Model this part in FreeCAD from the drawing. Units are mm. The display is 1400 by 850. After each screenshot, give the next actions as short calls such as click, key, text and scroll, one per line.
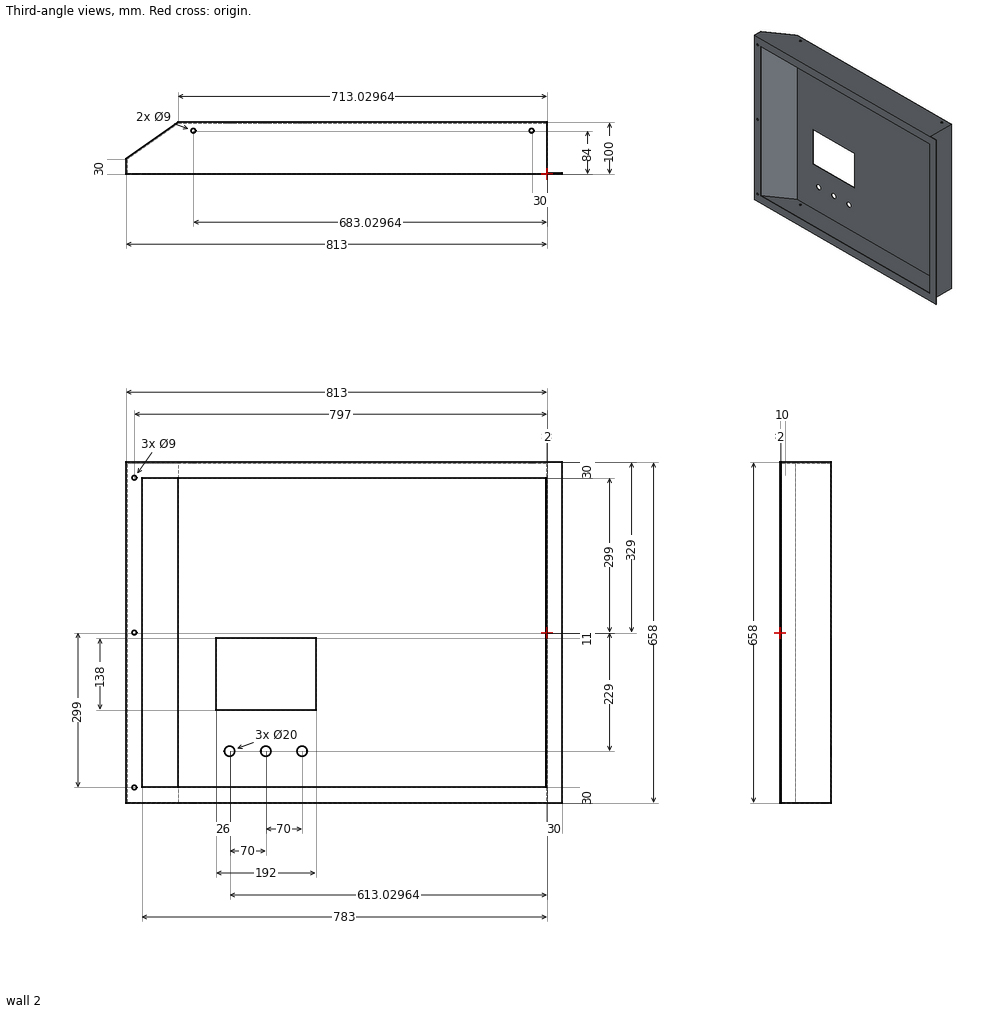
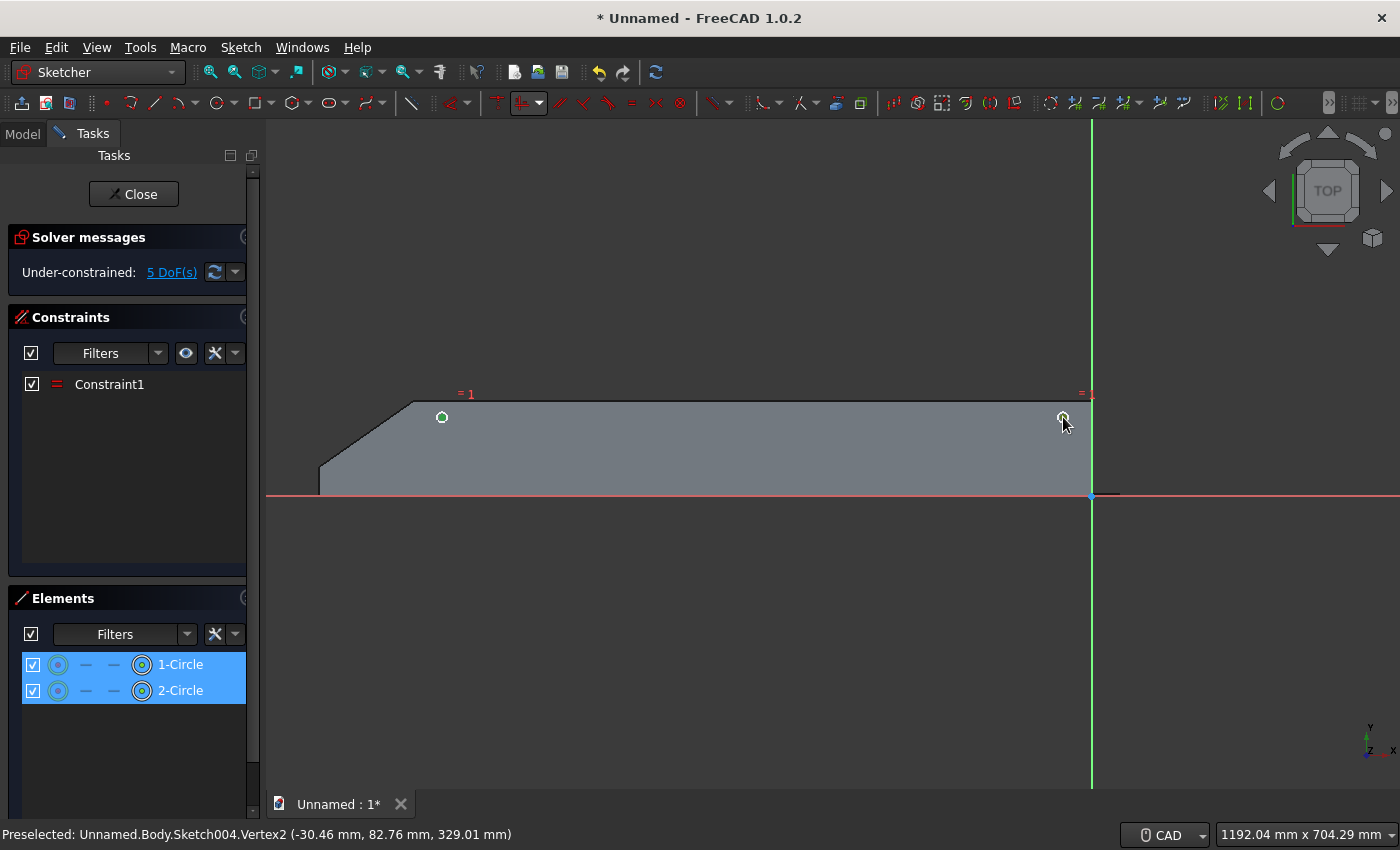
click(542, 104)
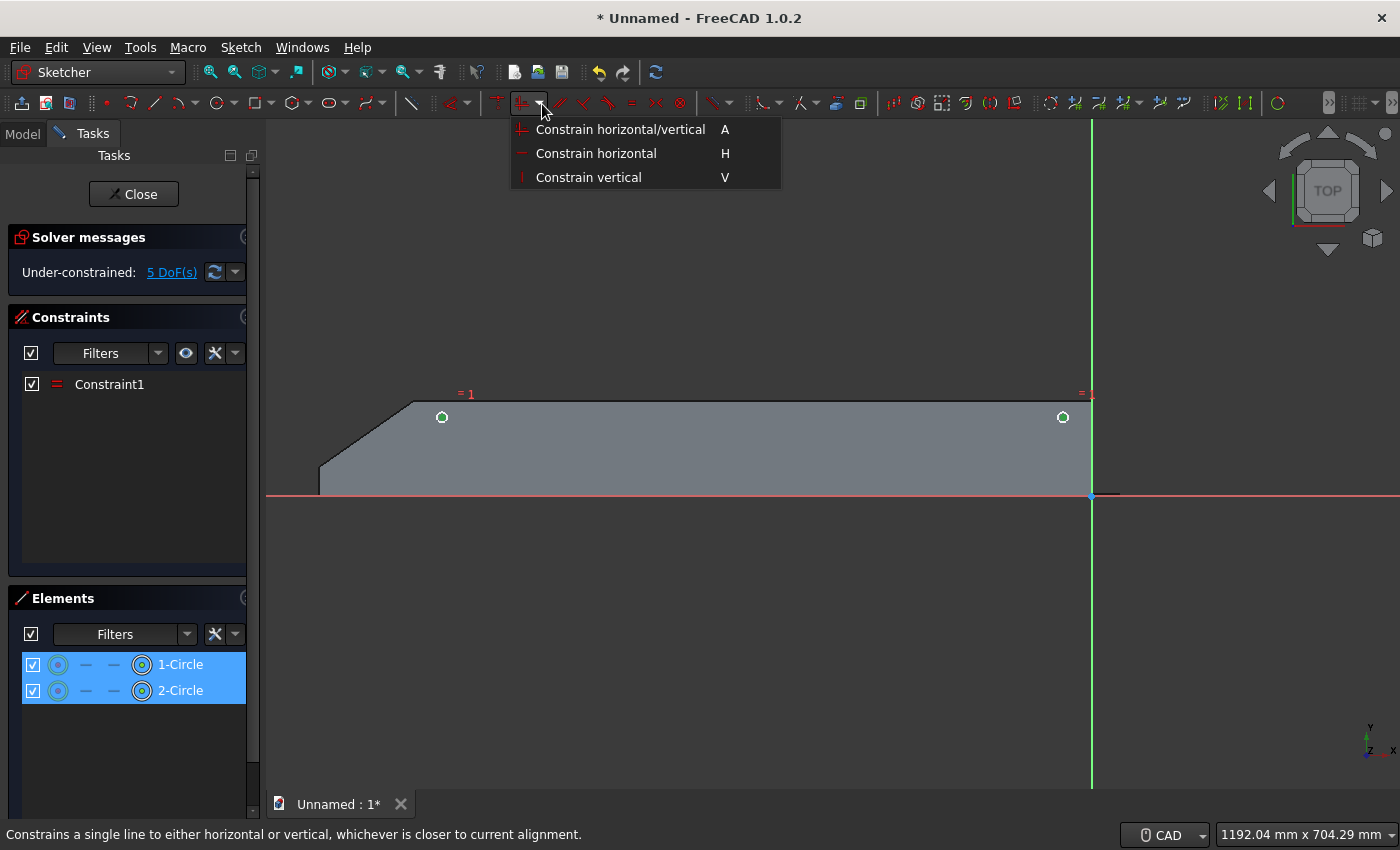
click(646, 153)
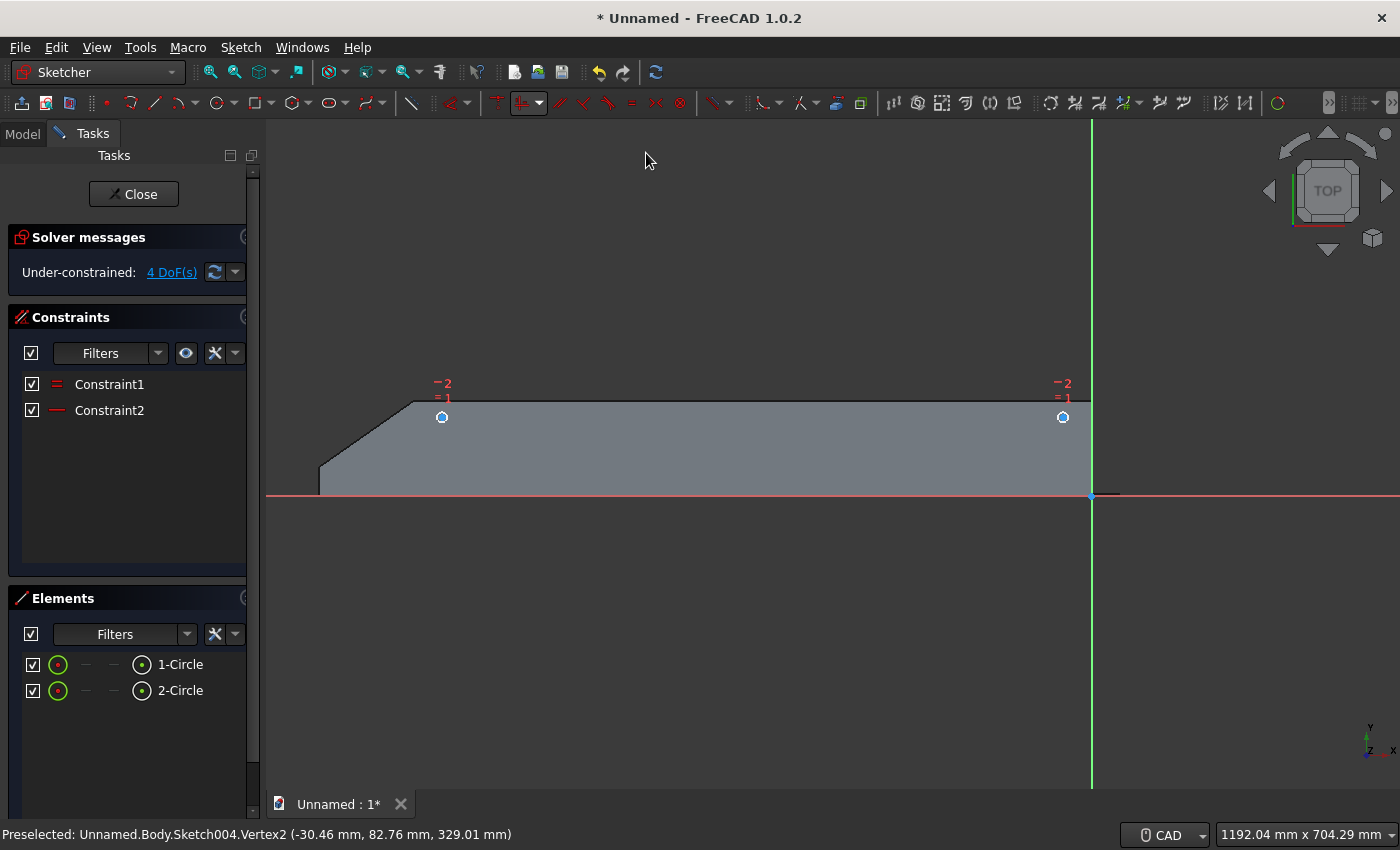
key(d)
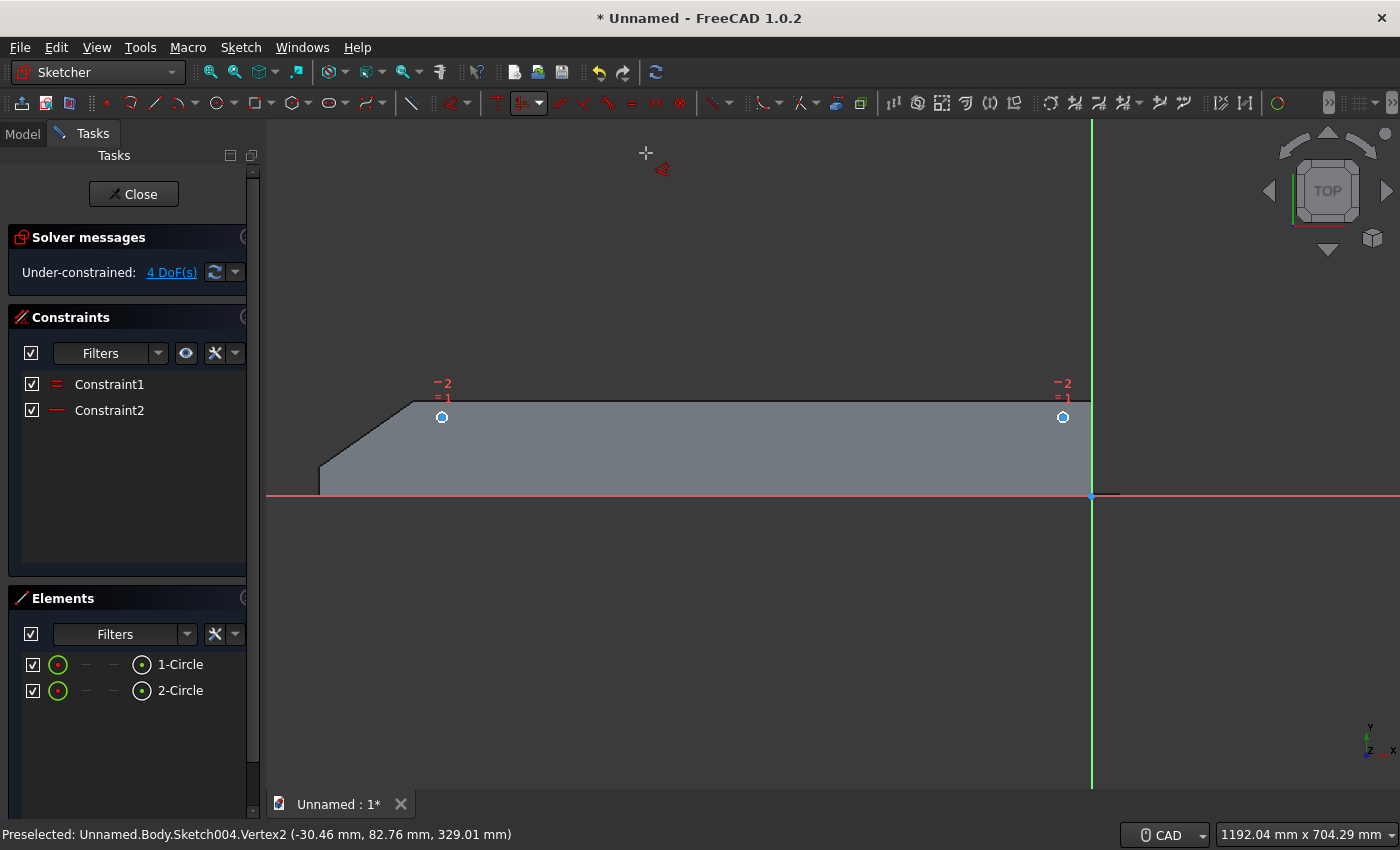
scroll(437, 417, up, 8)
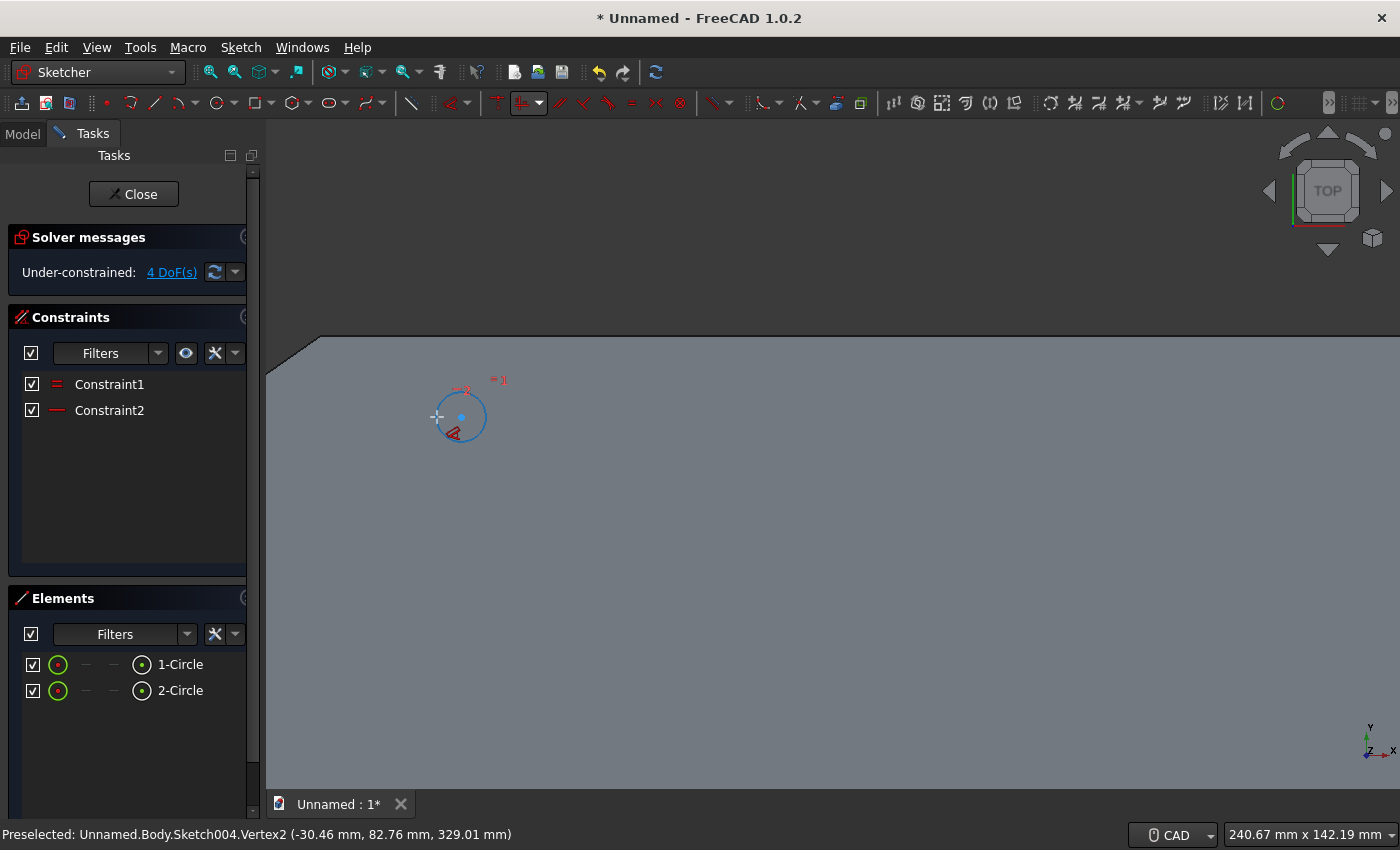
click(436, 416)
click(404, 415)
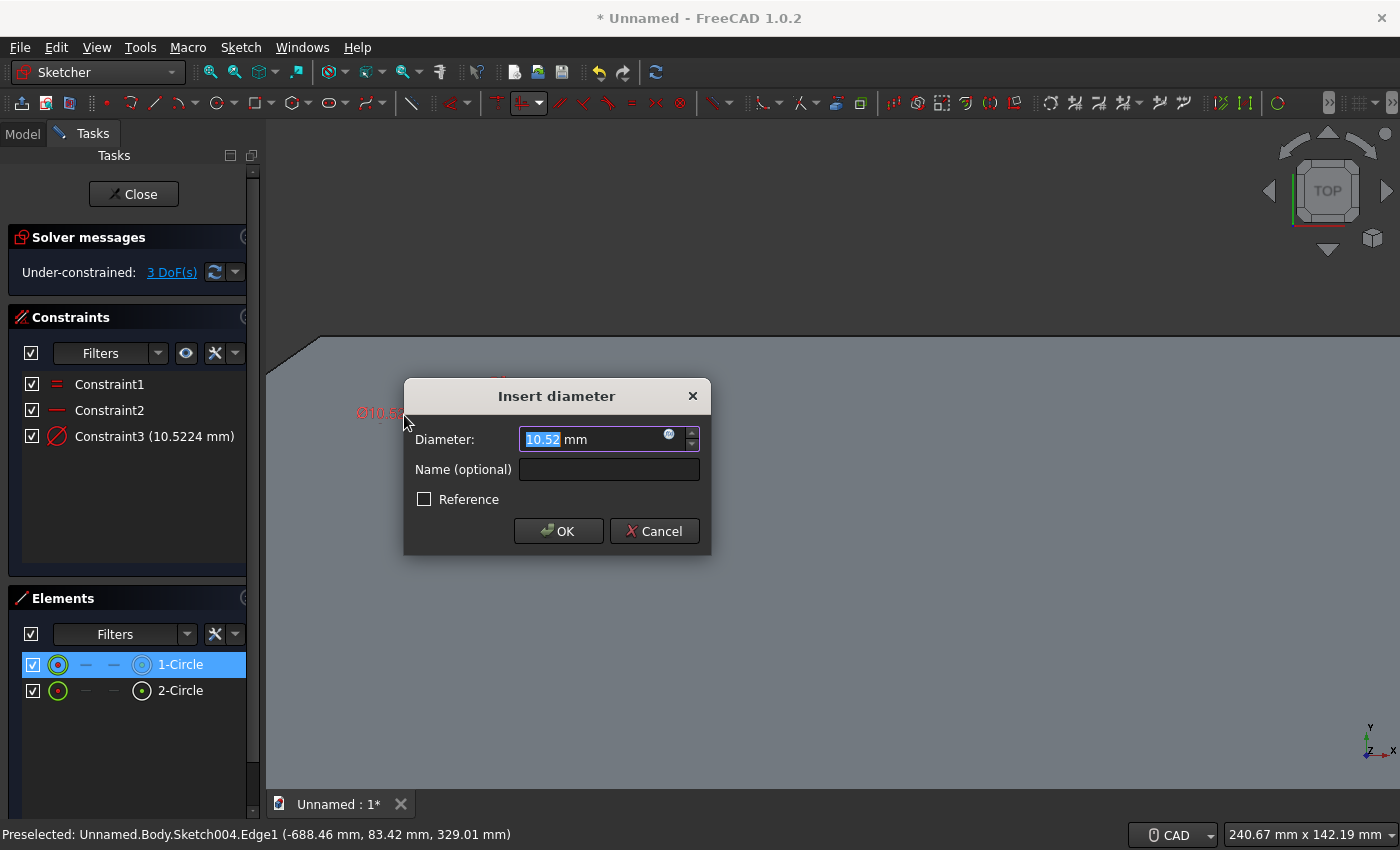
text(9)
key(Return)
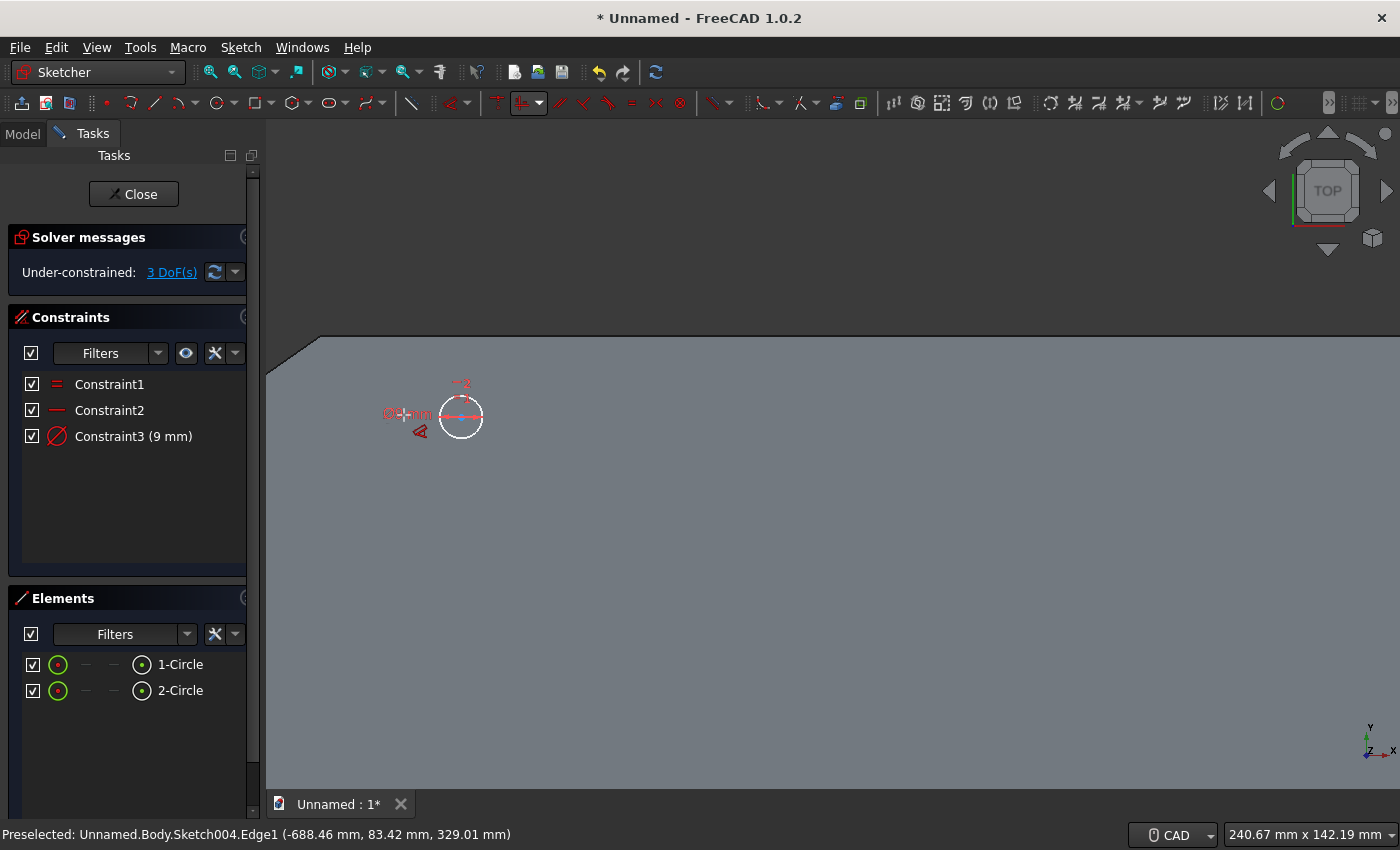
scroll(437, 417, down, 8)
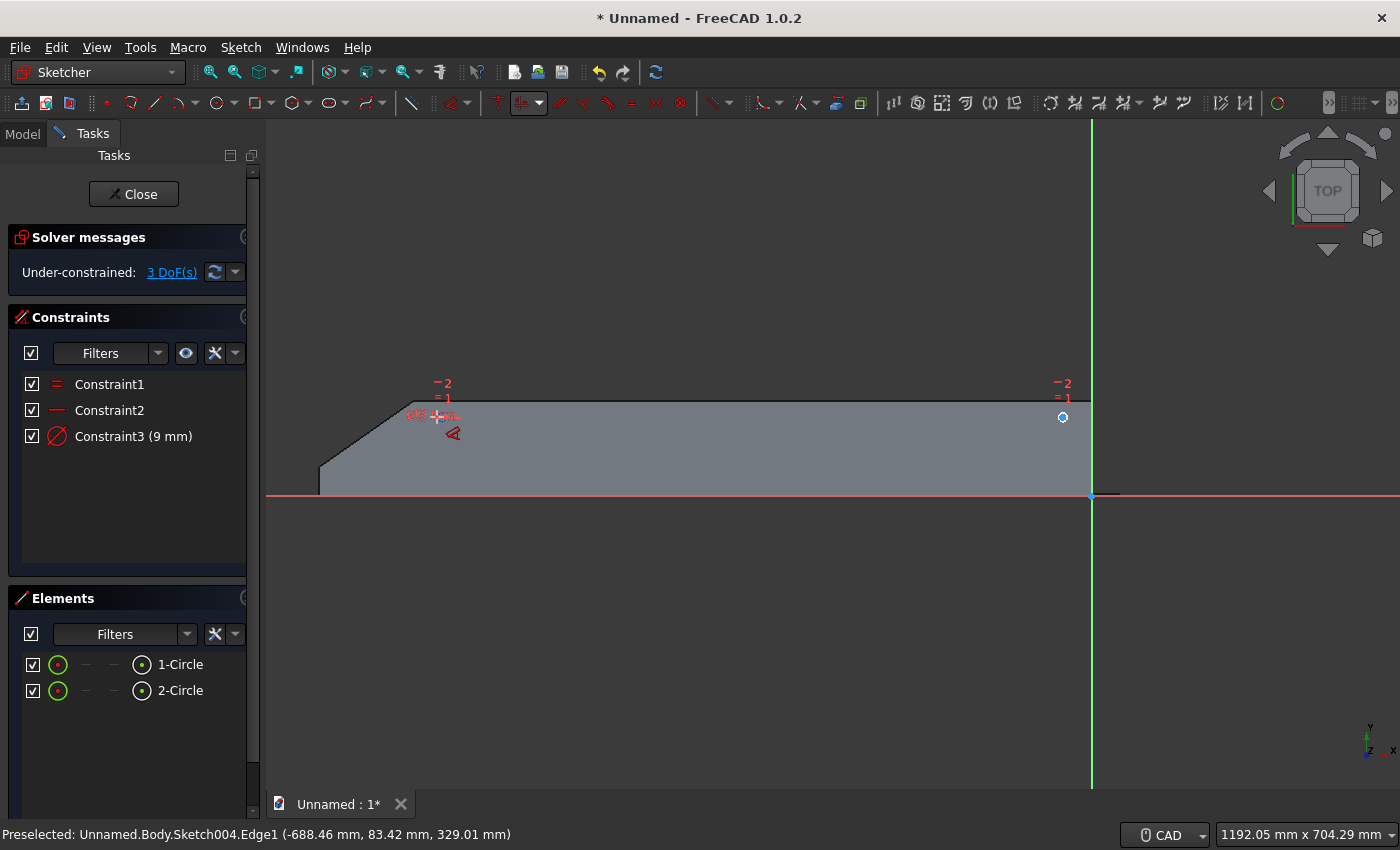
click(442, 417)
click(1126, 457)